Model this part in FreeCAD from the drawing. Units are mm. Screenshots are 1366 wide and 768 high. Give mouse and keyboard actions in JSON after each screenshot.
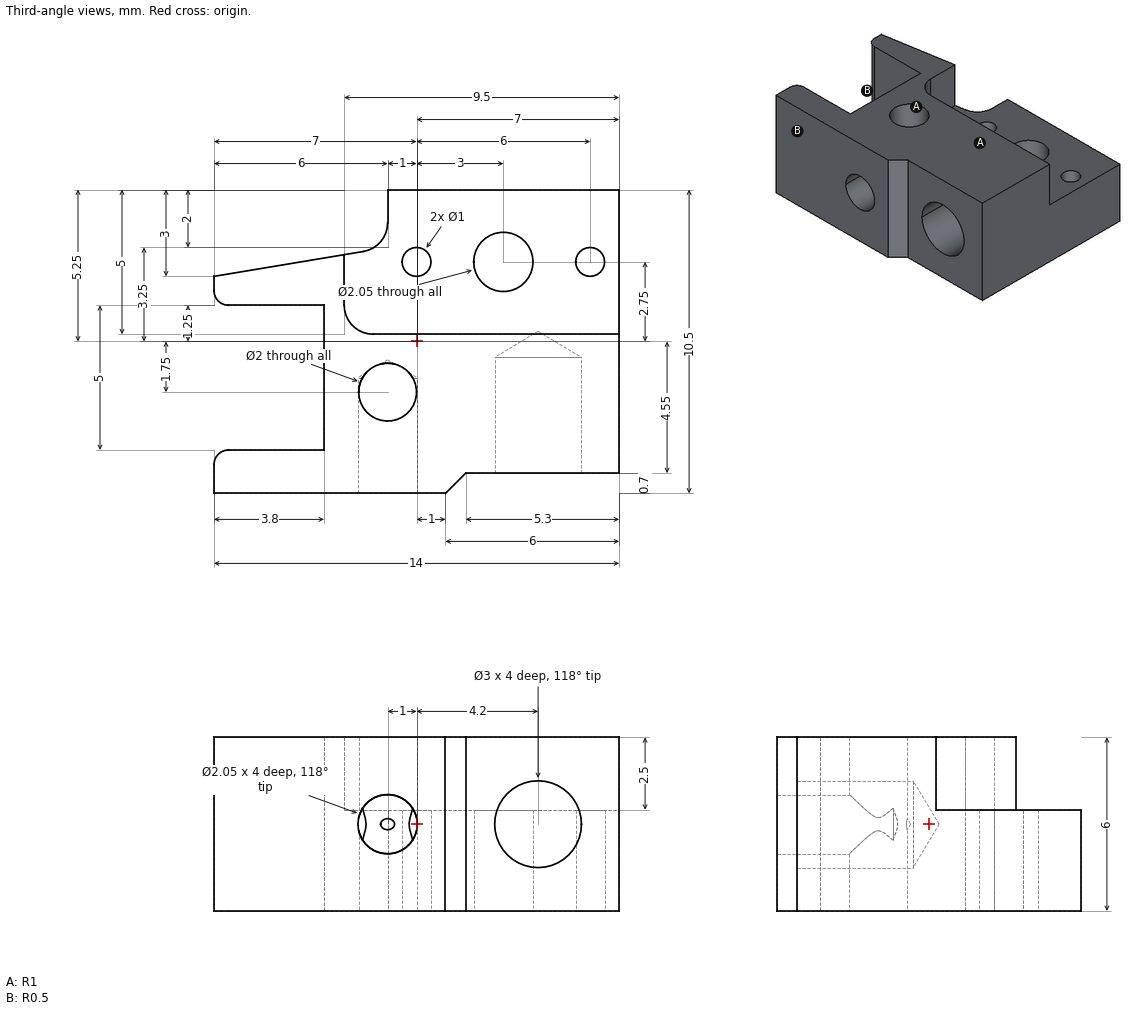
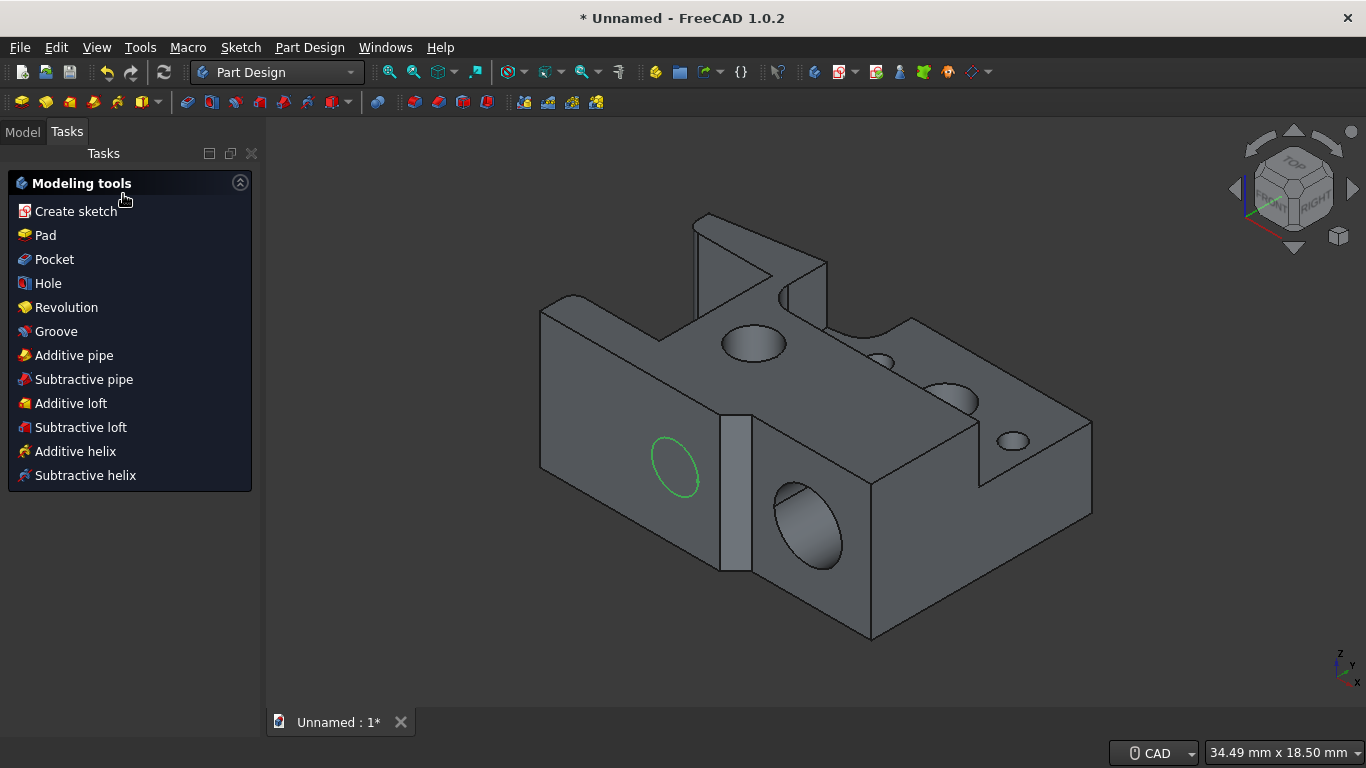
{"action": "left_click", "coordinate": [212, 102]}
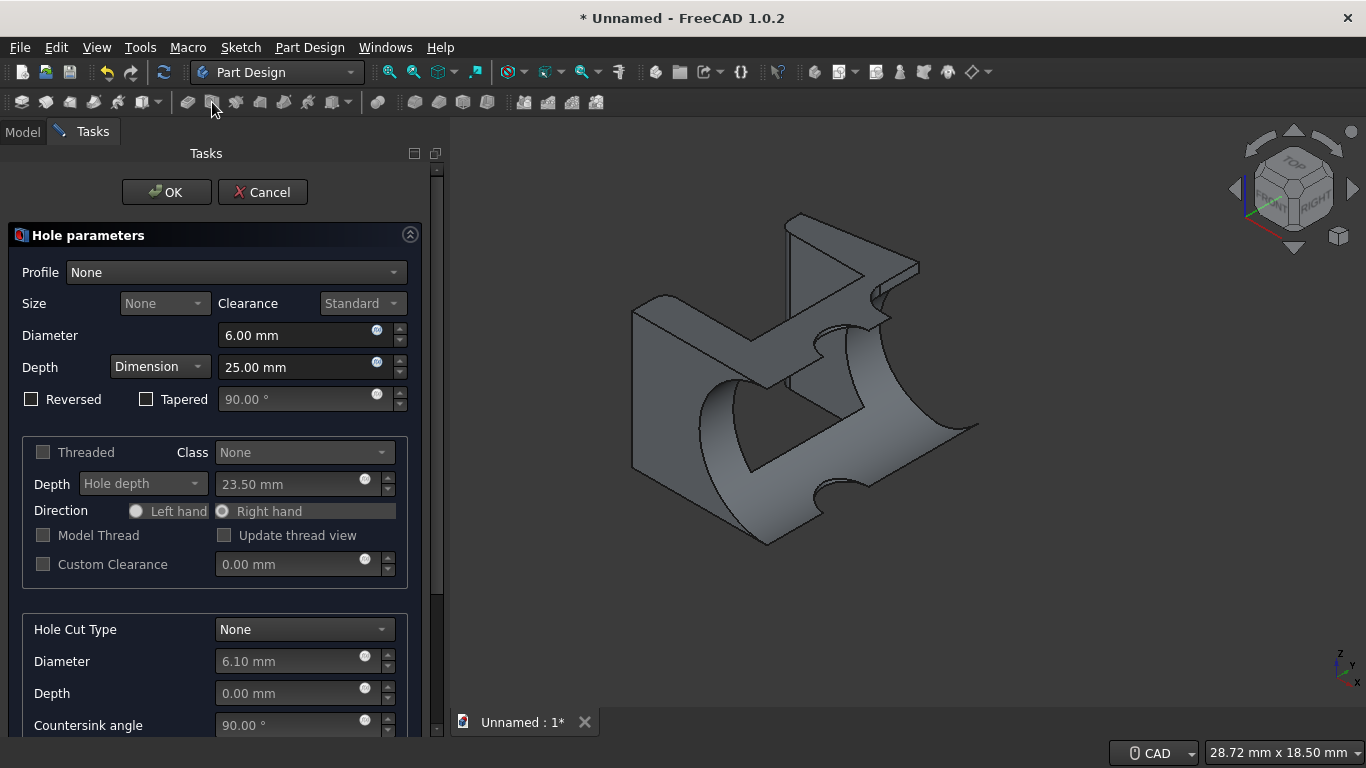
{"action": "triple_click", "coordinate": [305, 335]}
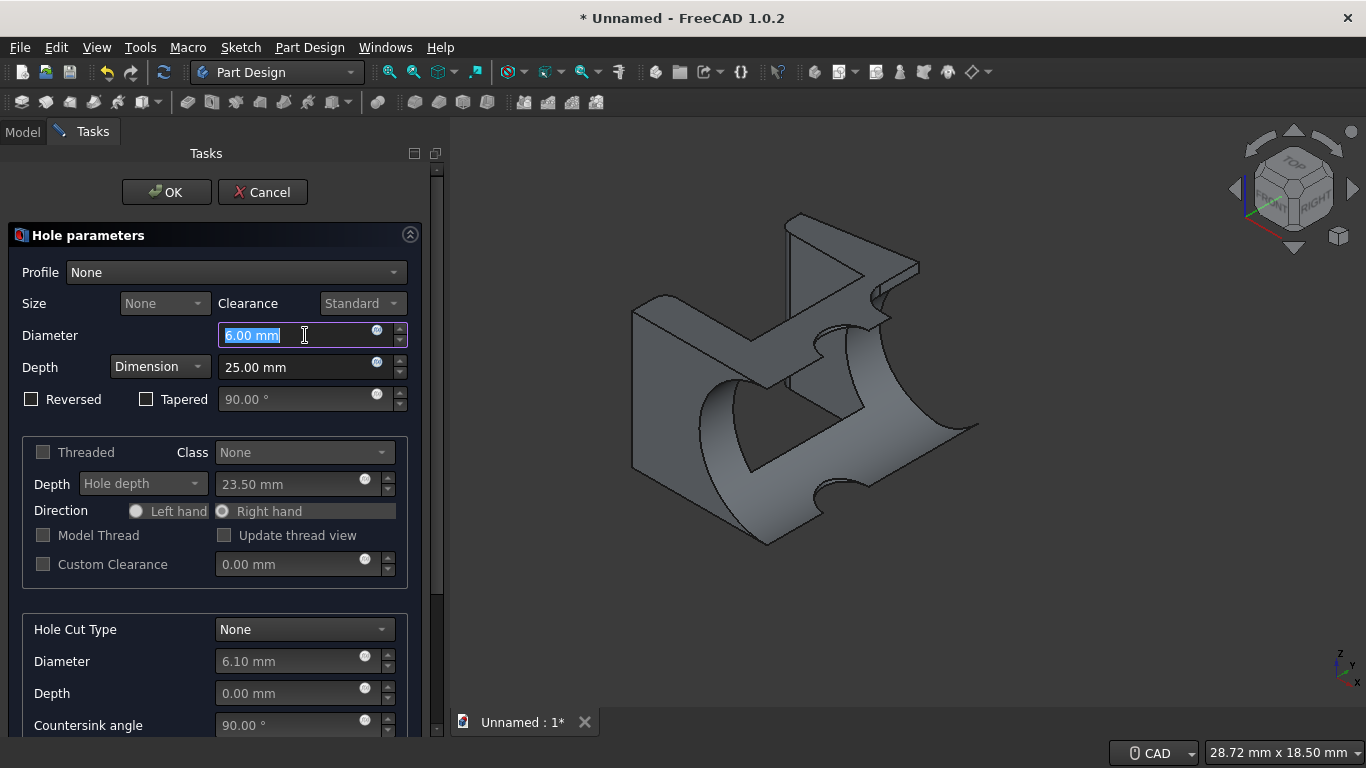
{"action": "type", "text": "2.05"}
{"action": "key", "text": "Tab"}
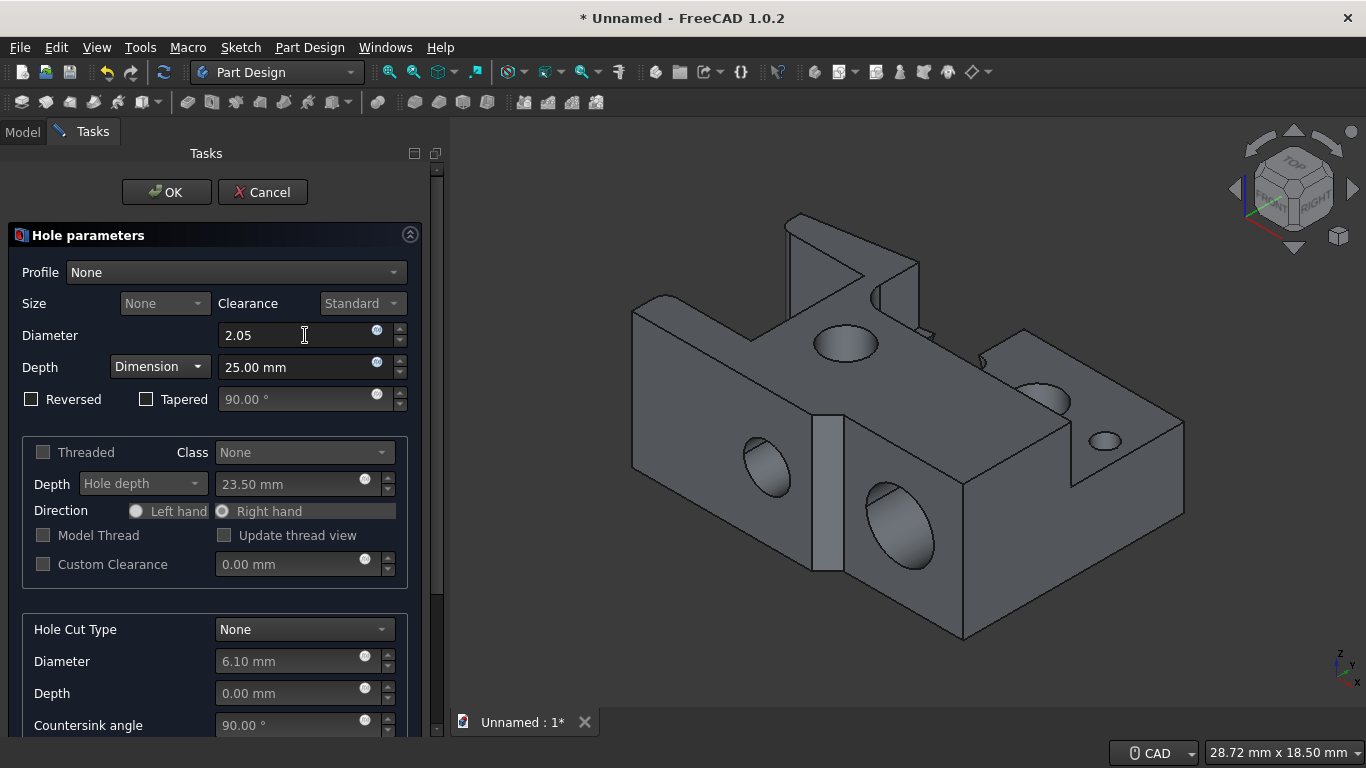
{"action": "triple_click", "coordinate": [305, 367]}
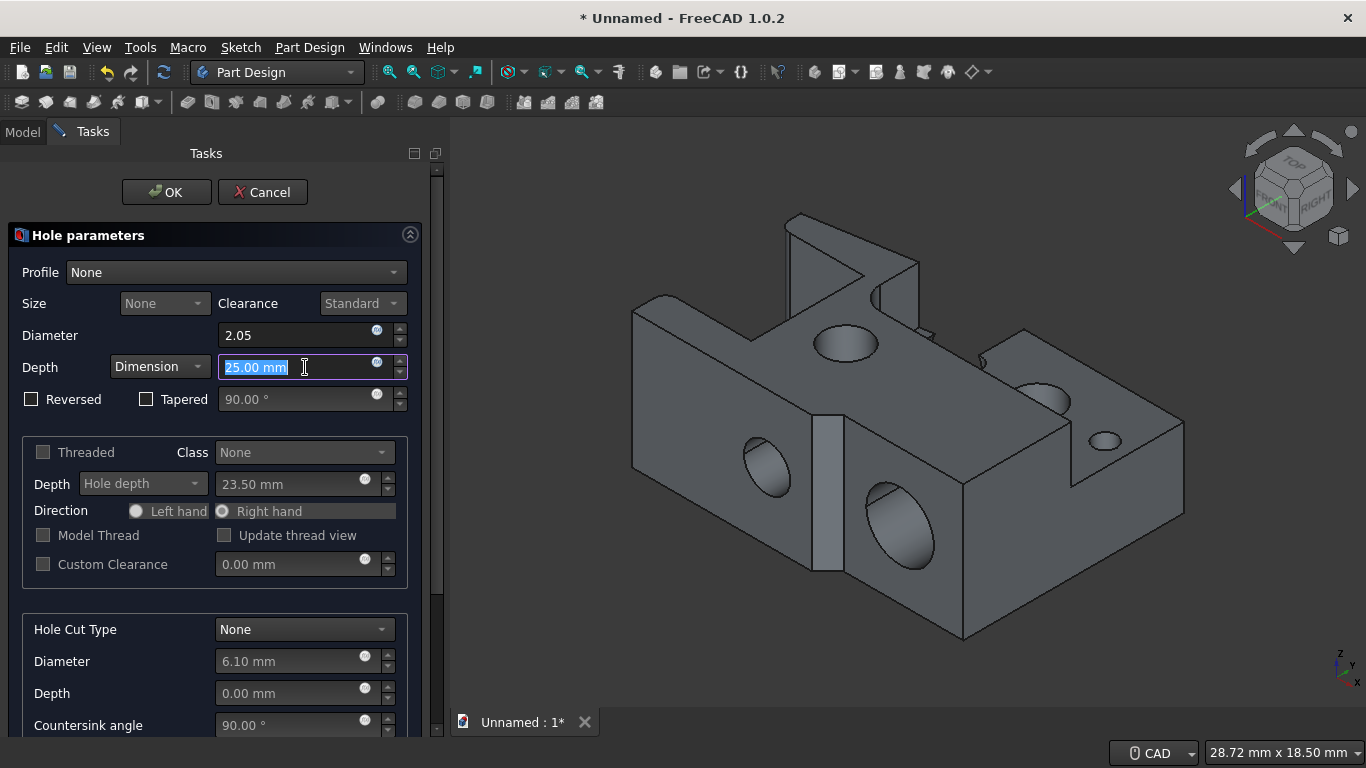
{"action": "type", "text": "4"}
{"action": "key", "text": "Tab"}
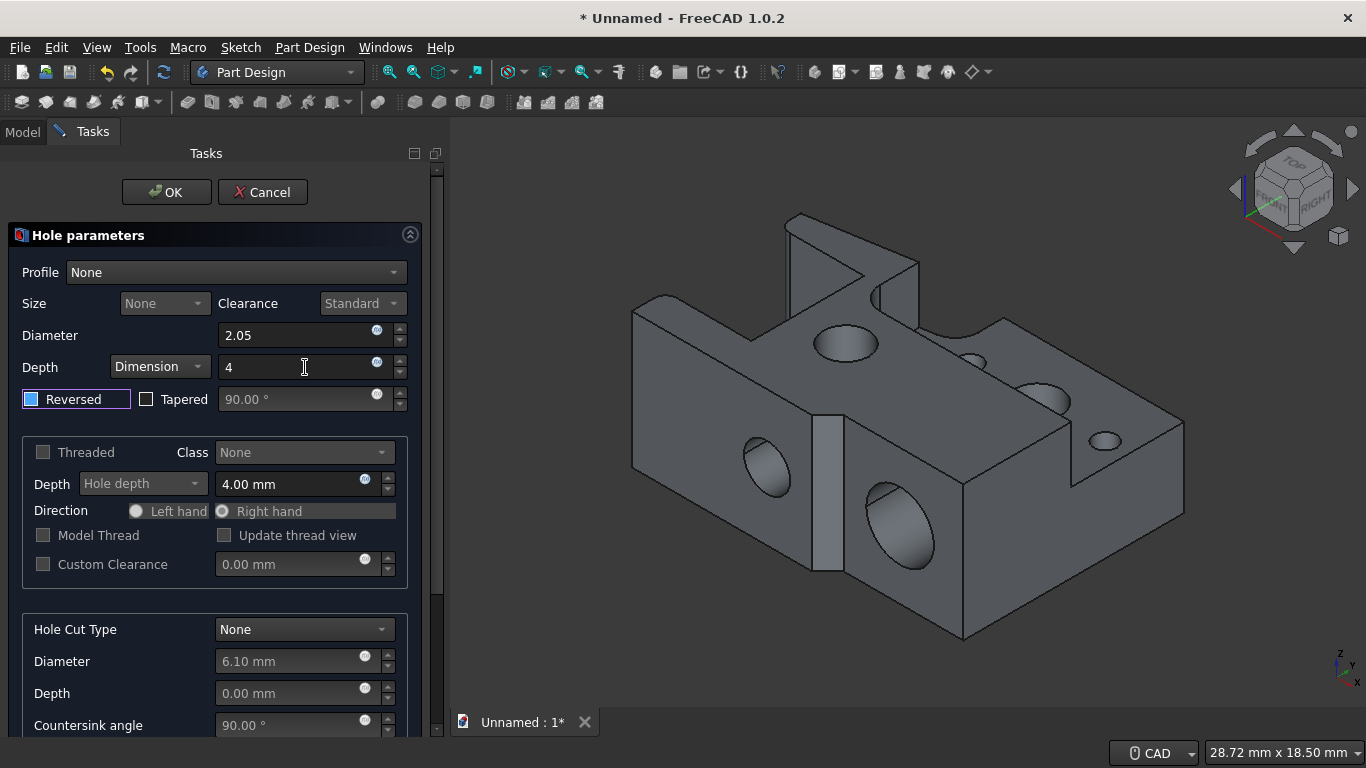
{"action": "left_click", "coordinate": [167, 192]}